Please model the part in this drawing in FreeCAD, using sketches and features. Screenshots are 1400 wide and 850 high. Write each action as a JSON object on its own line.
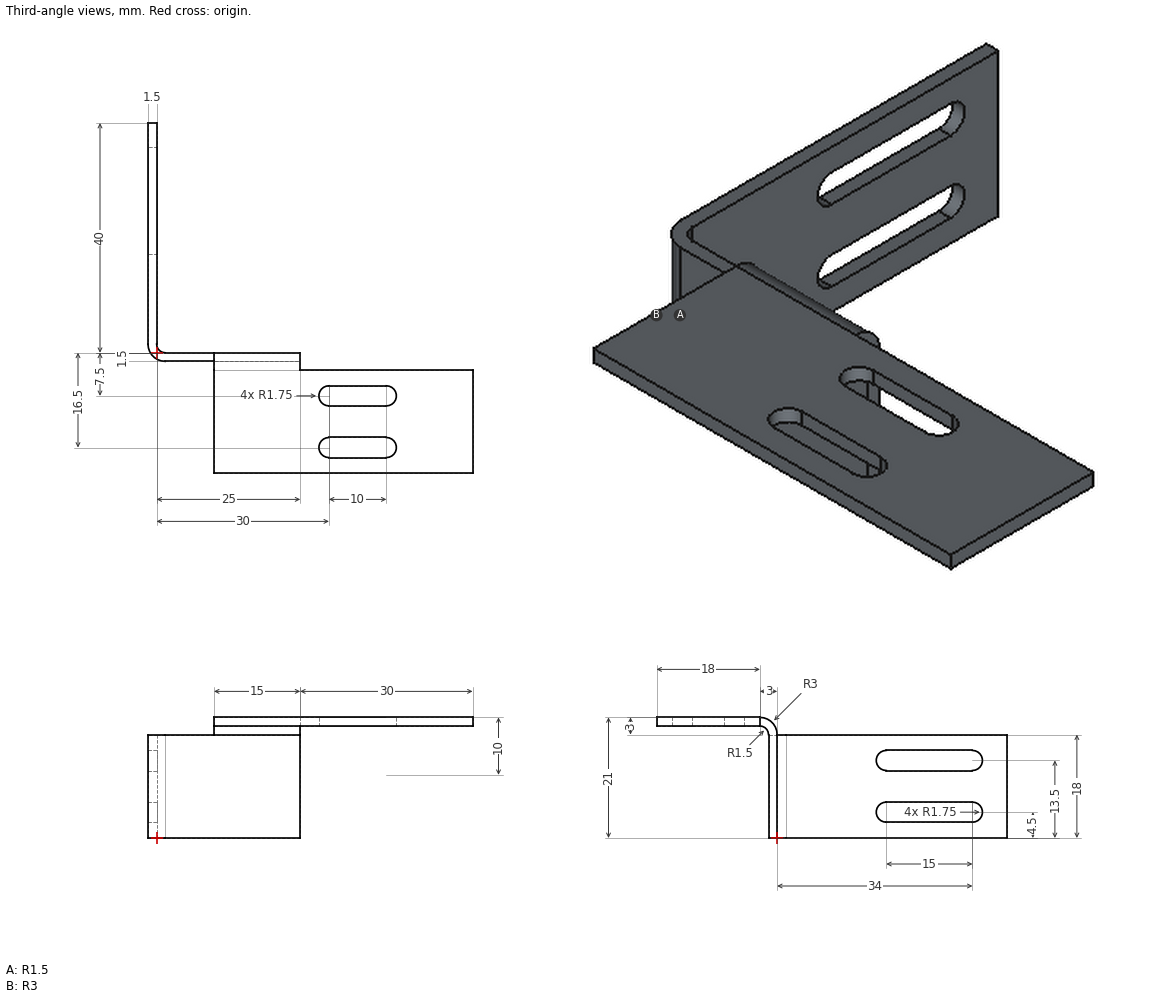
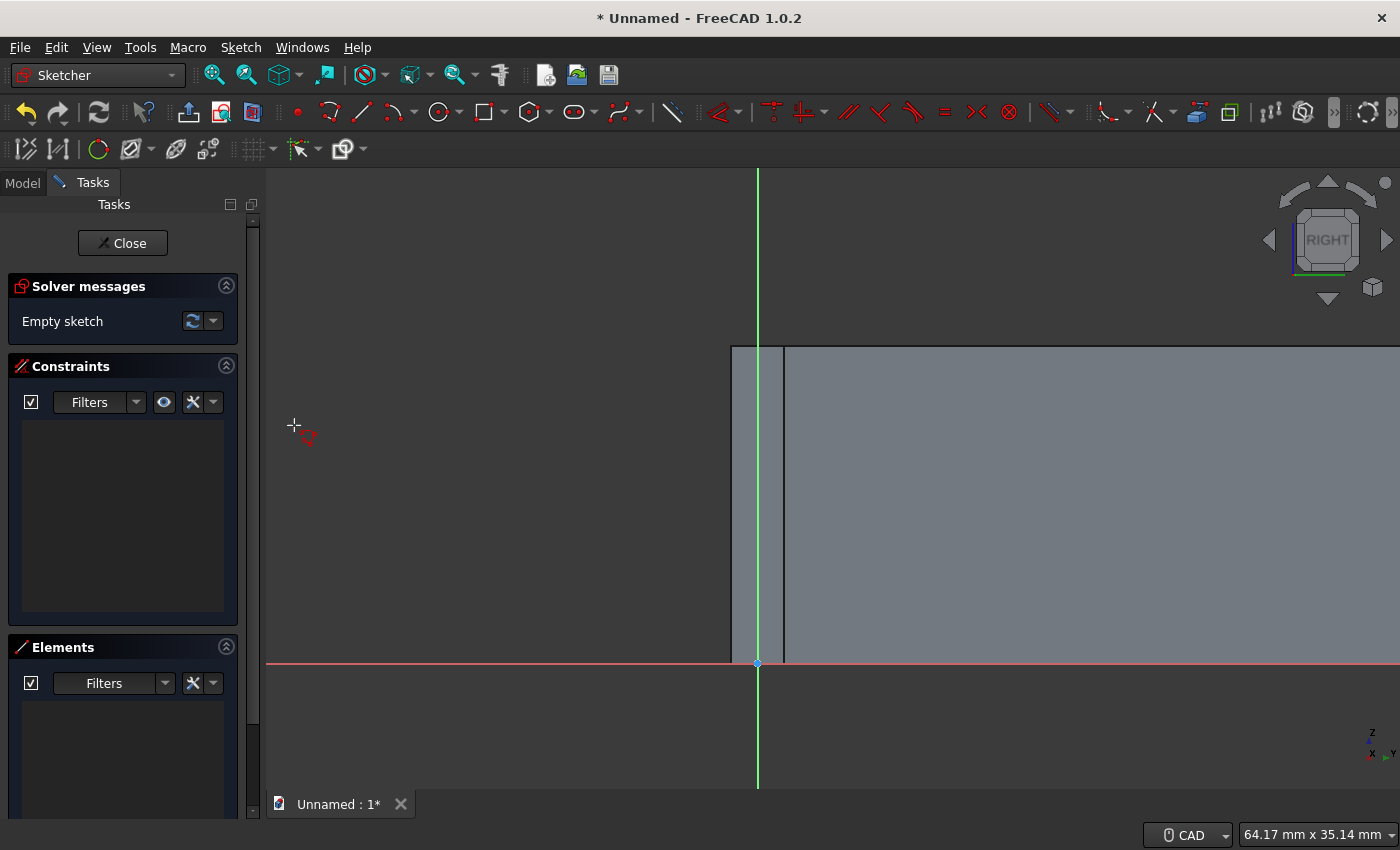
{"action": "left_click", "coordinate": [705, 293]}
{"action": "left_click", "coordinate": [387, 293]}
{"action": "left_click", "coordinate": [387, 319]}
{"action": "left_click", "coordinate": [705, 319]}
{"action": "right_click", "coordinate": [705, 319]}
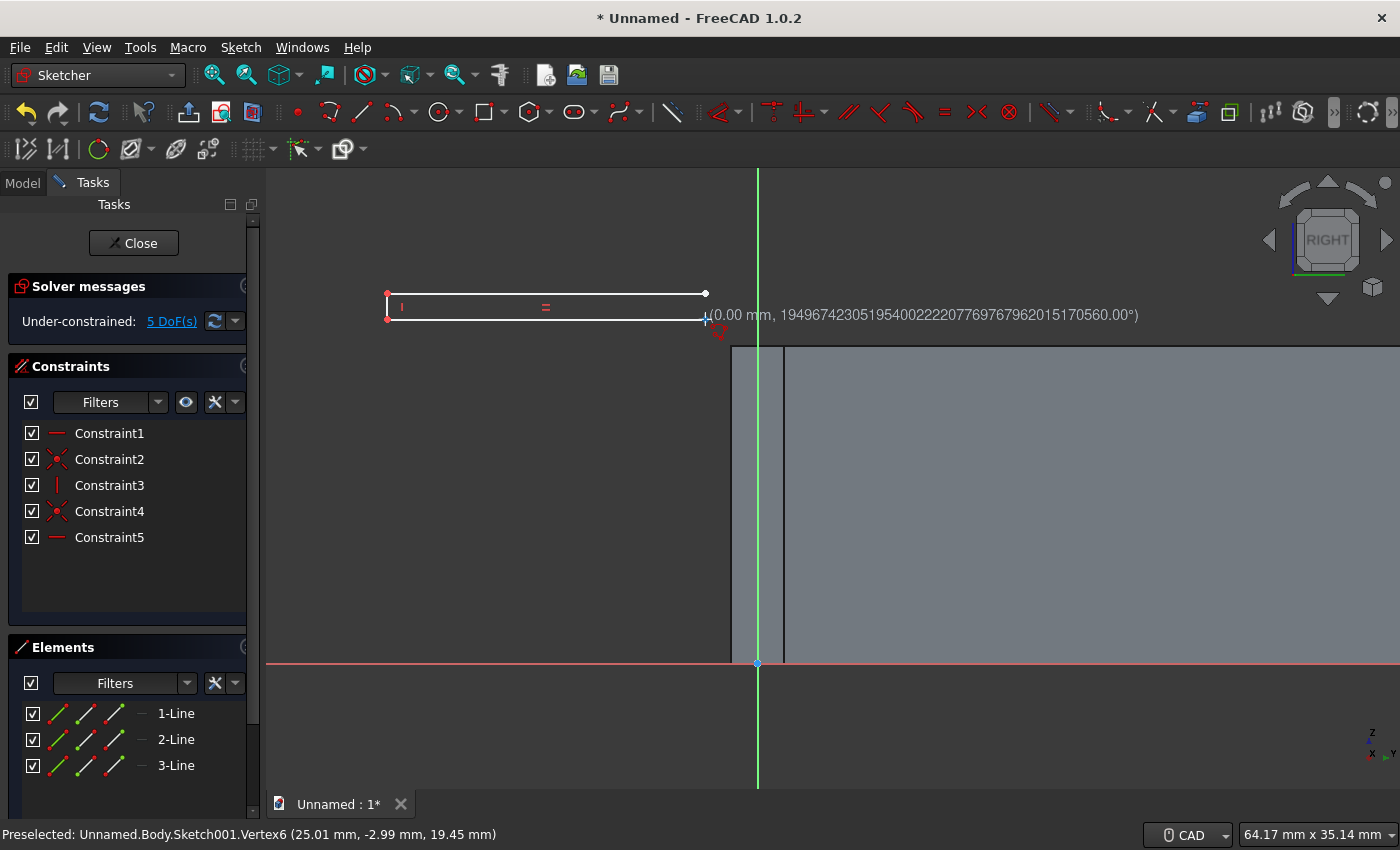
{"action": "key", "text": "g l"}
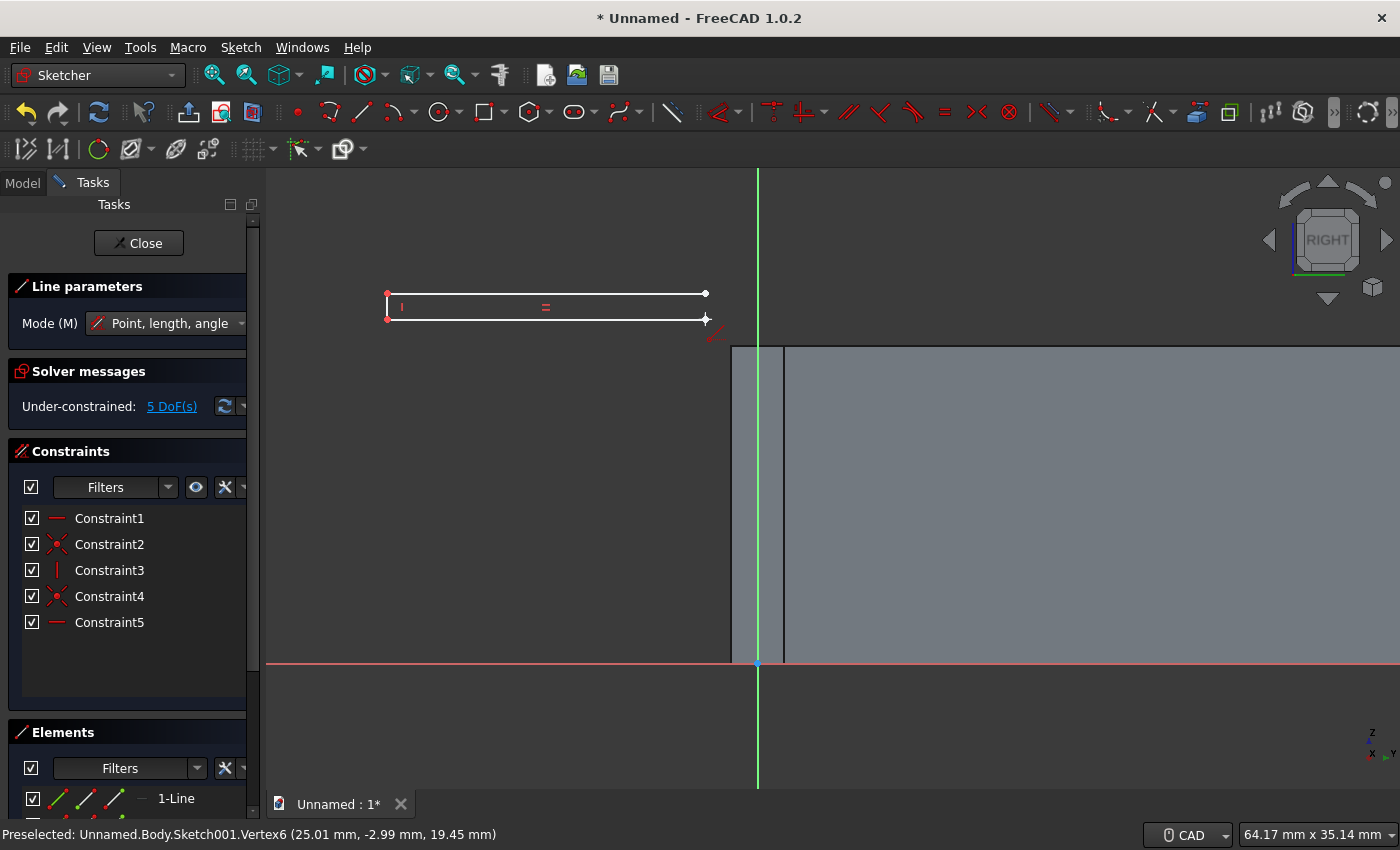
{"action": "left_click", "coordinate": [731, 346]}
{"action": "left_click", "coordinate": [758, 346]}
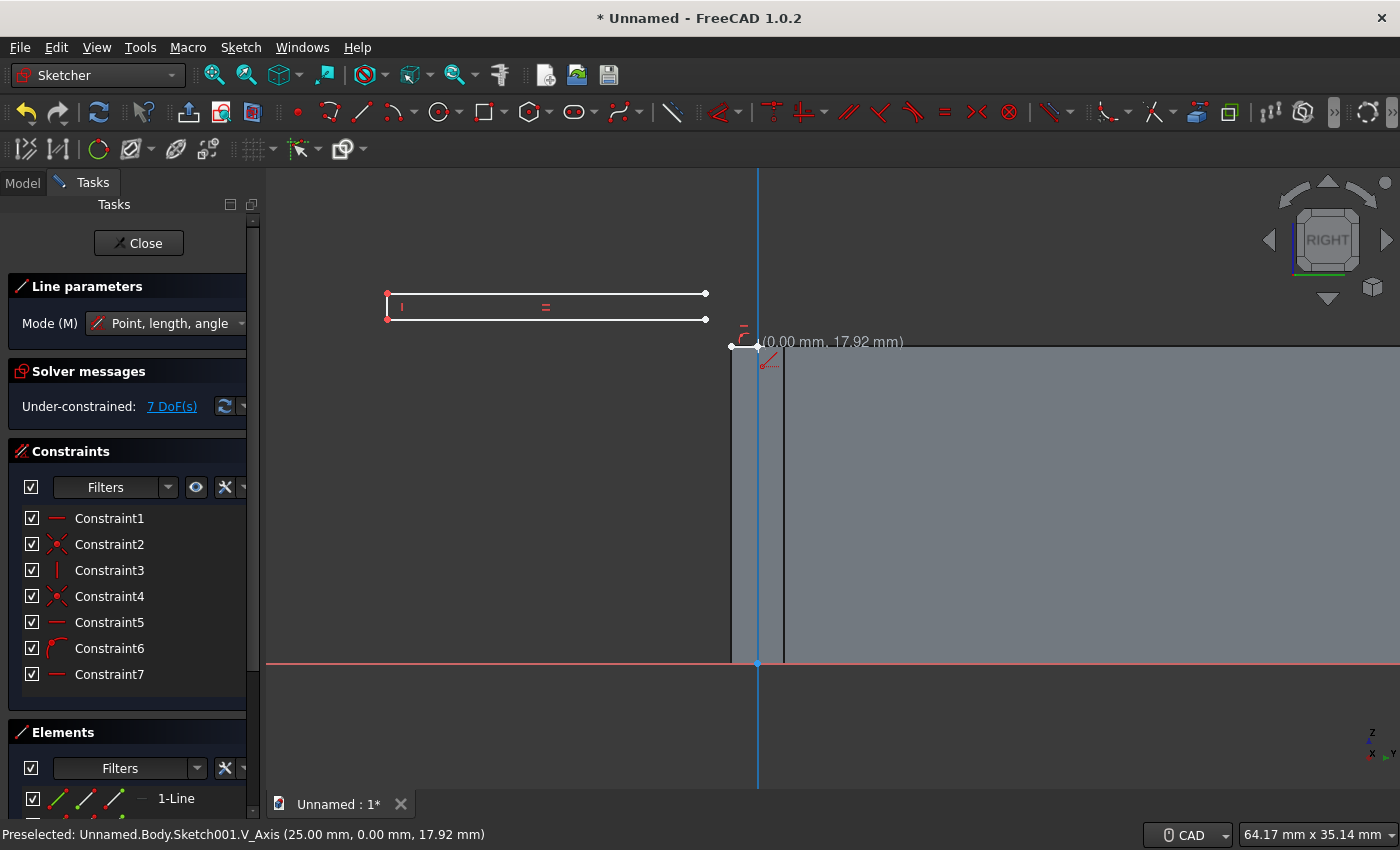
{"action": "key", "text": "g 3 a"}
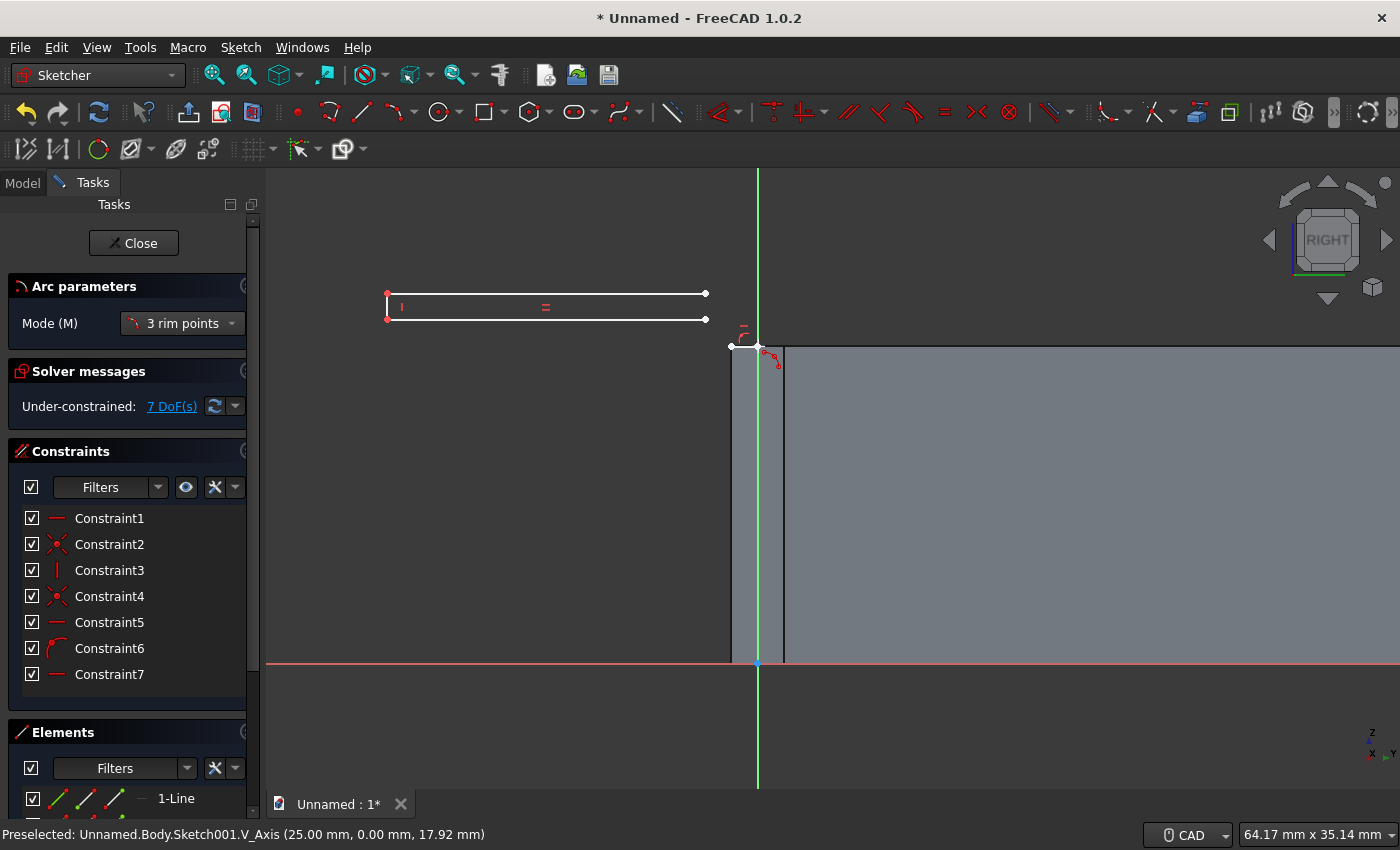
{"action": "left_click", "coordinate": [705, 320]}
{"action": "left_click", "coordinate": [731, 347]}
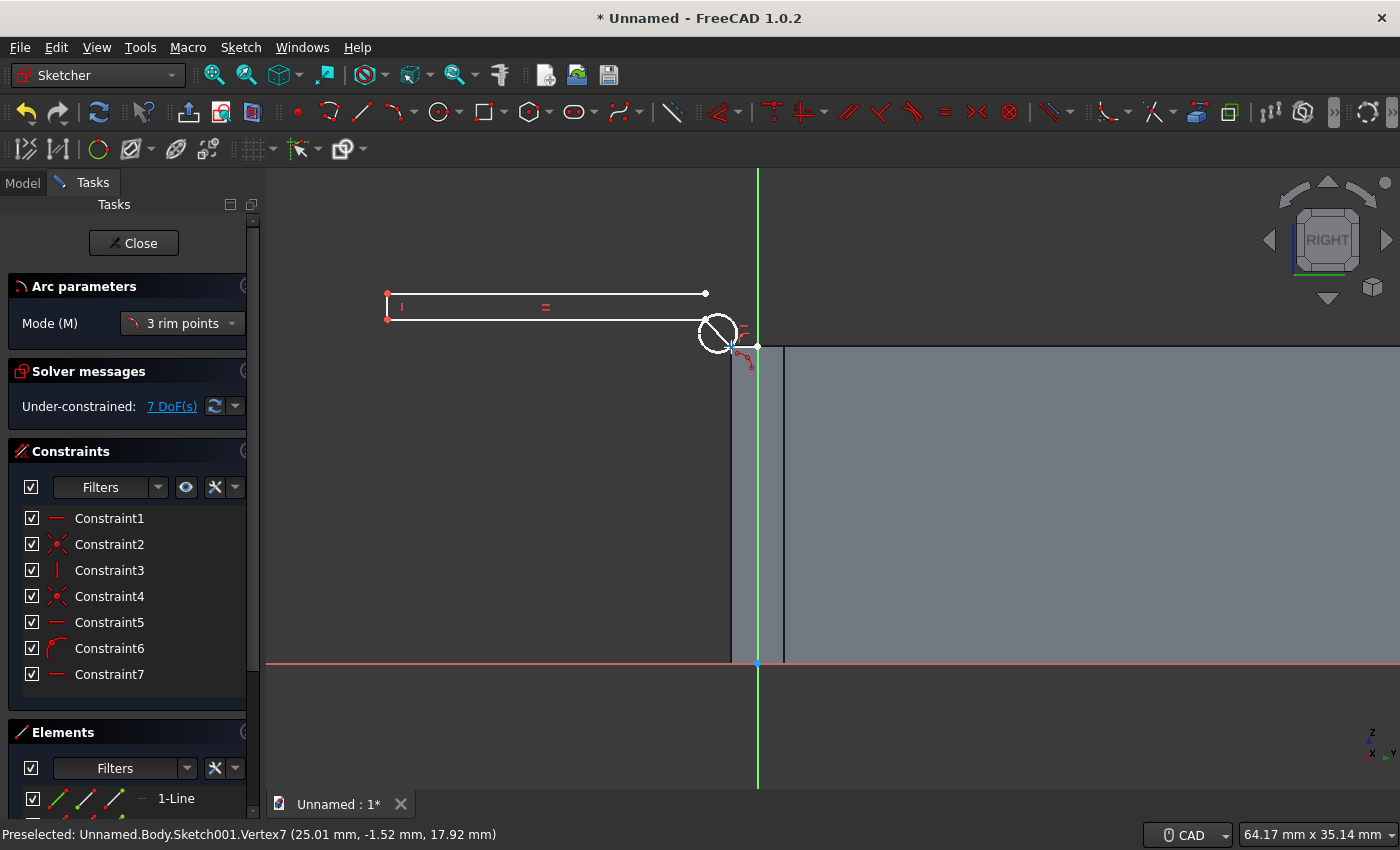
{"action": "scroll", "coordinate": [724, 327], "scroll_direction": "up", "scroll_amount": 4}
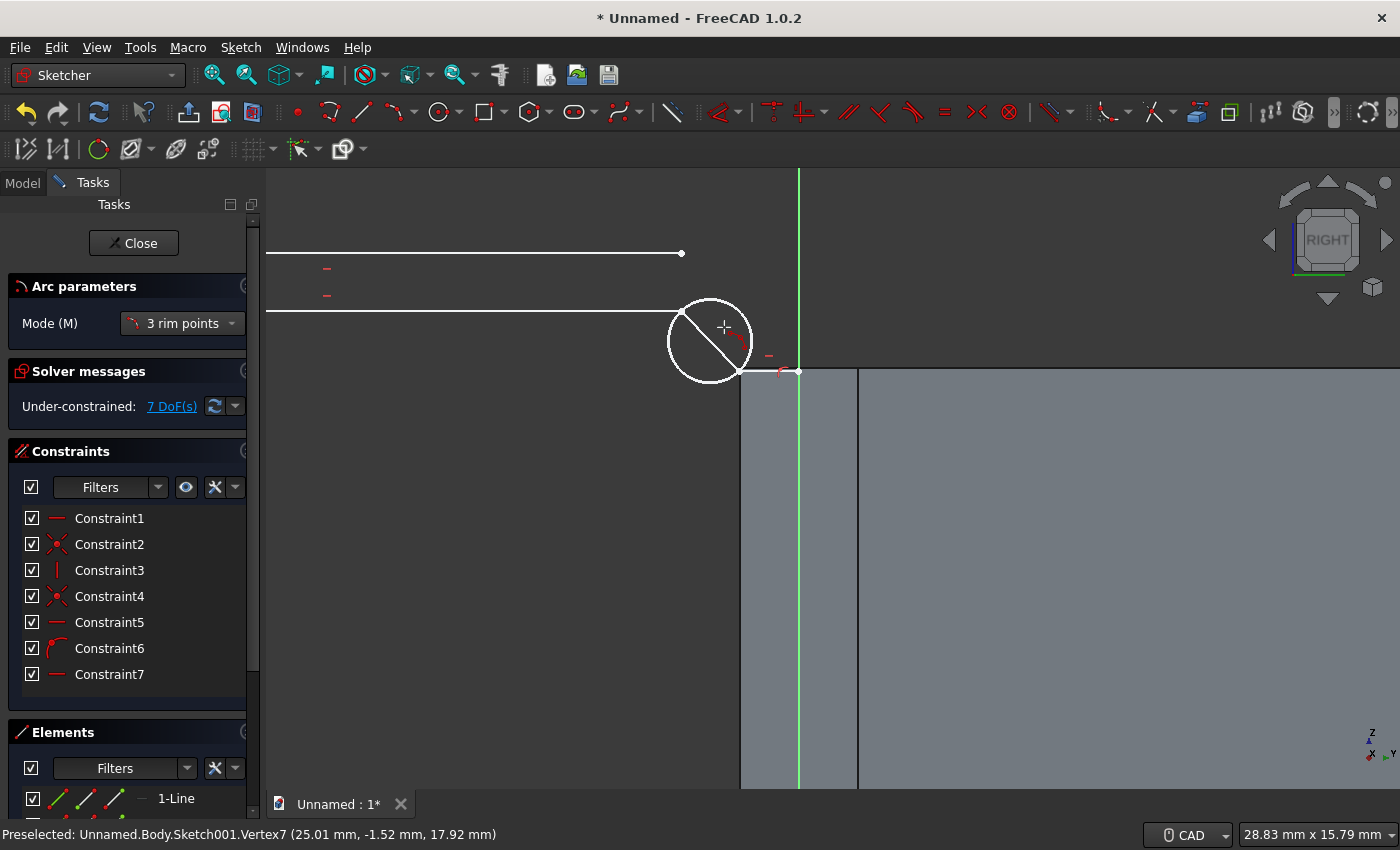
{"action": "left_click", "coordinate": [723, 326]}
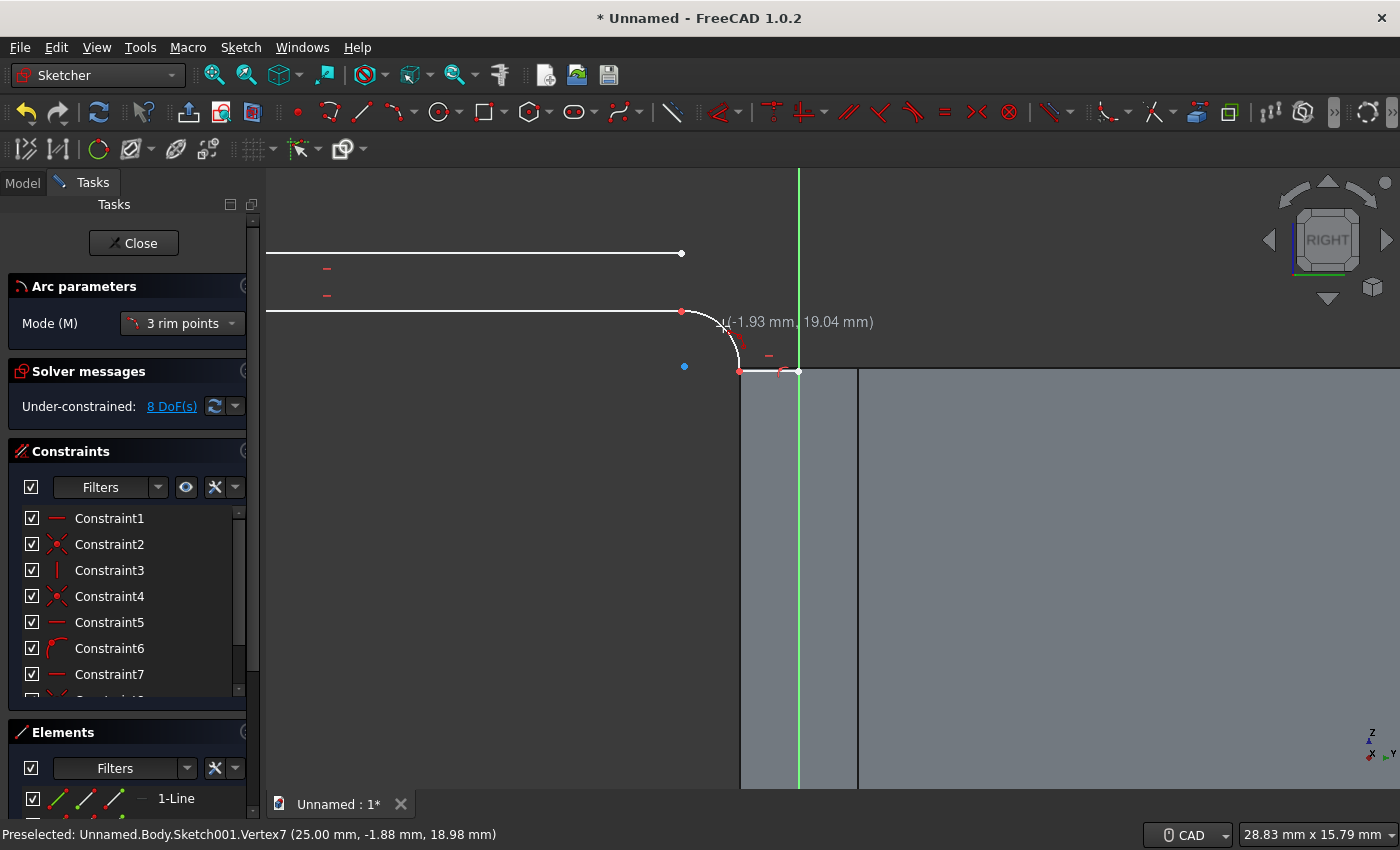
{"action": "left_click", "coordinate": [799, 371]}
{"action": "left_click", "coordinate": [681, 253]}
{"action": "left_click", "coordinate": [764, 285]}
{"action": "key", "text": "Escape"}